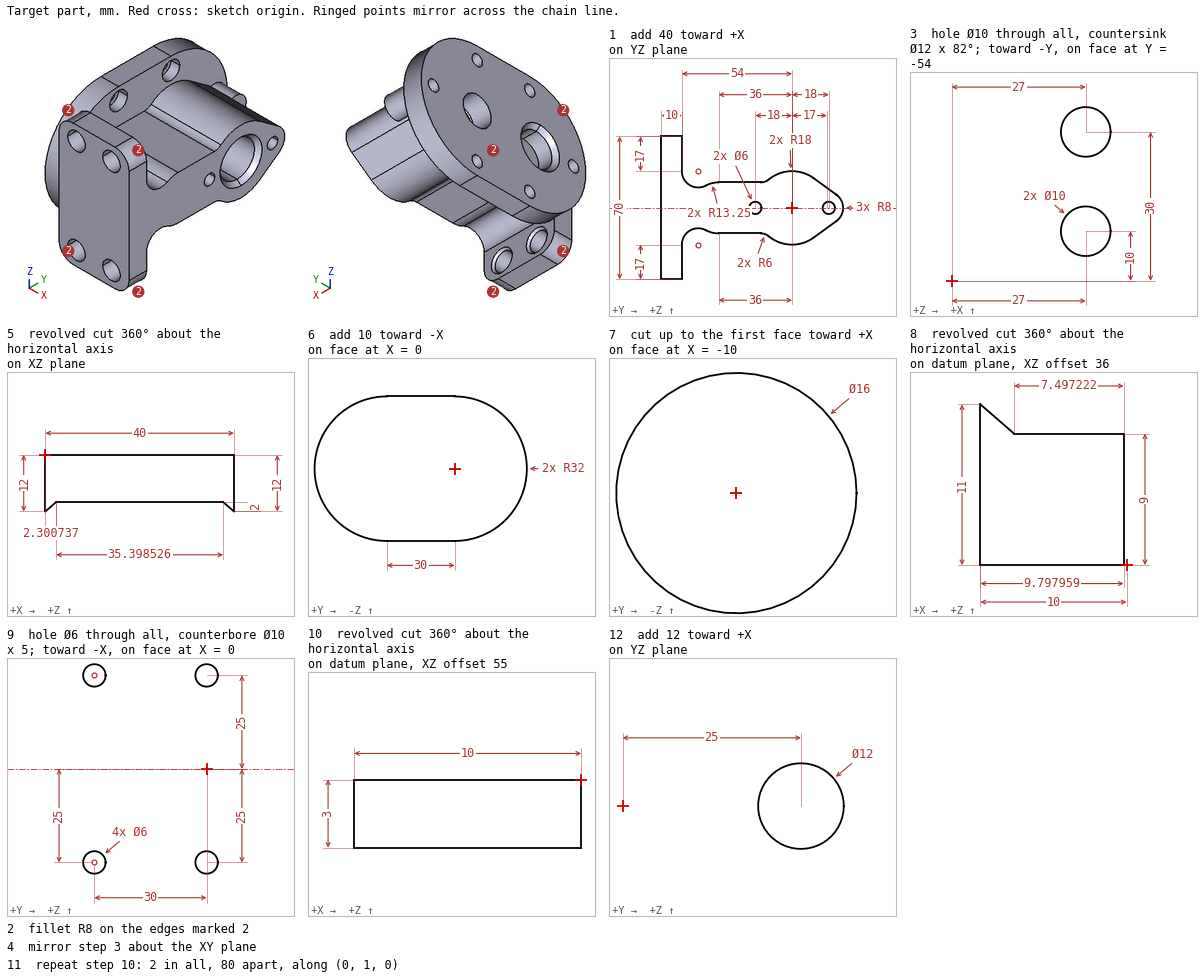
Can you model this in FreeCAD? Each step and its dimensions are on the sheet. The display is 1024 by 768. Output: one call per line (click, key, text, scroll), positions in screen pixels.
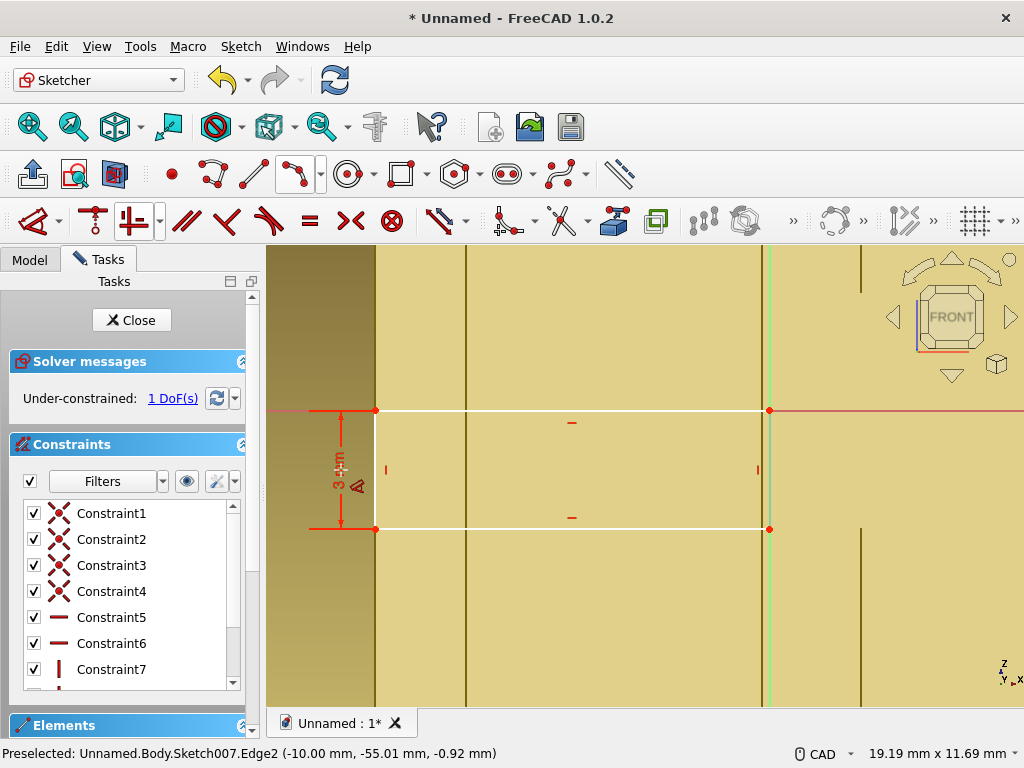
click(651, 411)
click(572, 377)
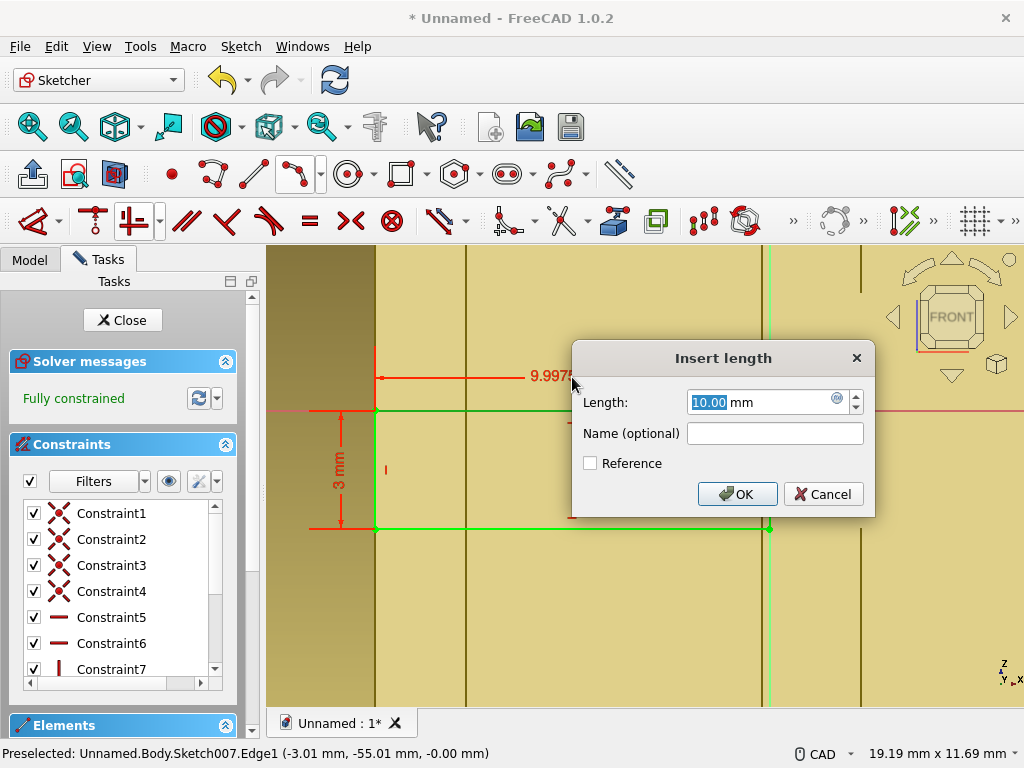
text(10)
key(Return)
key(Escape)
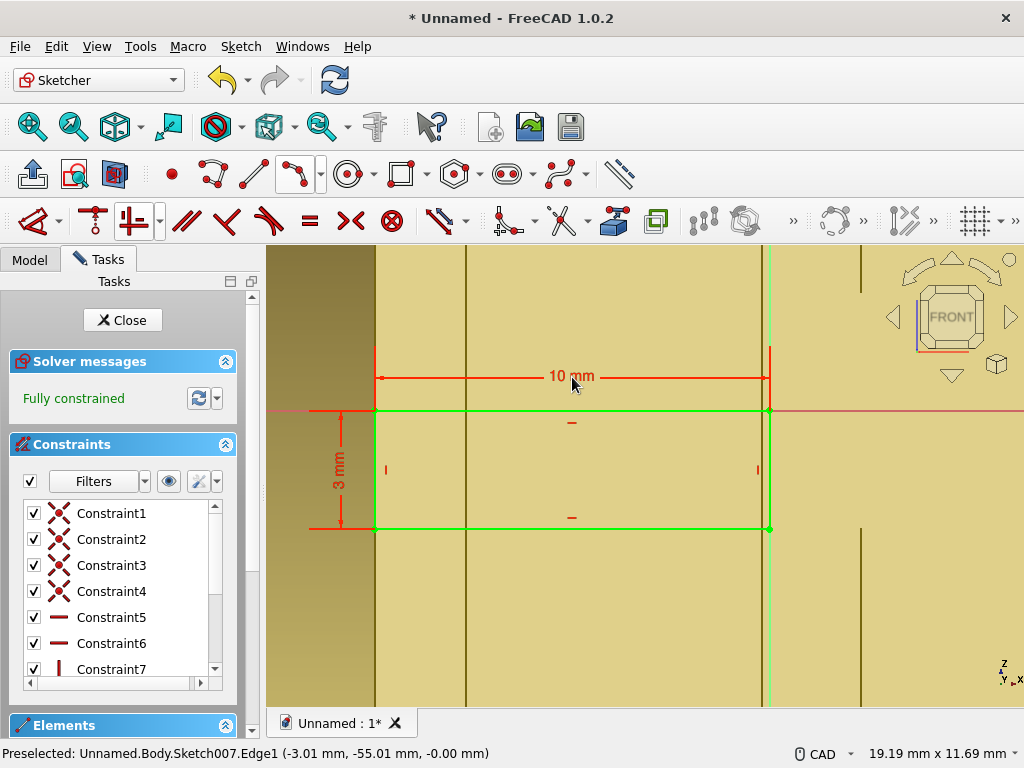
click(123, 320)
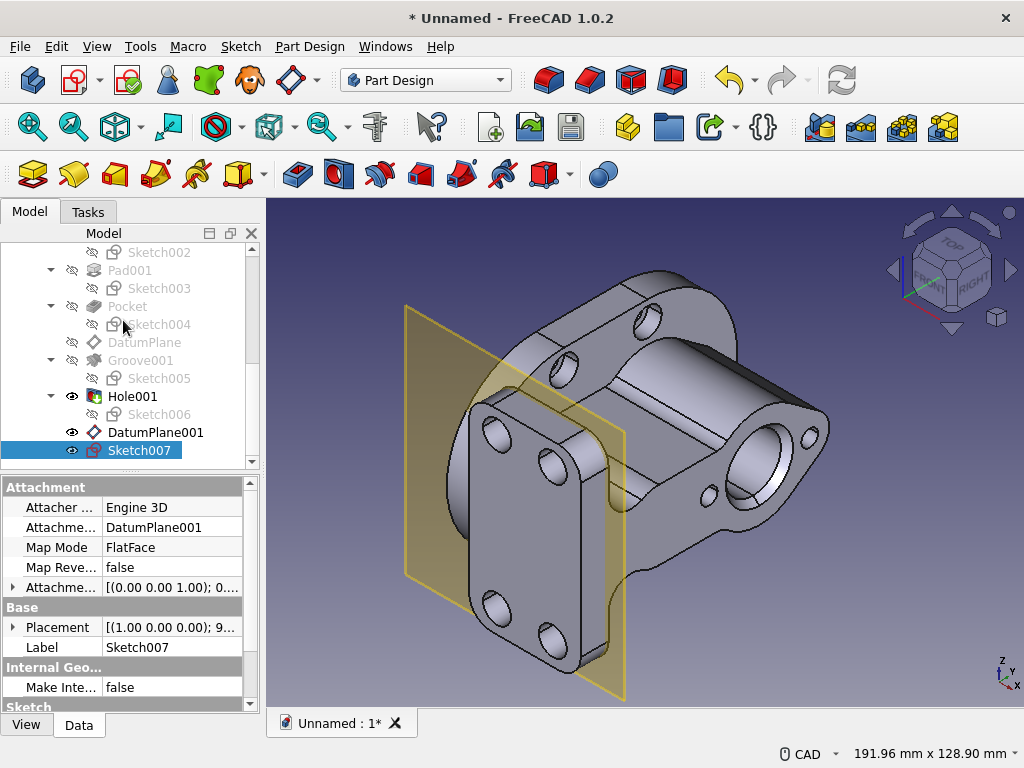
click(380, 174)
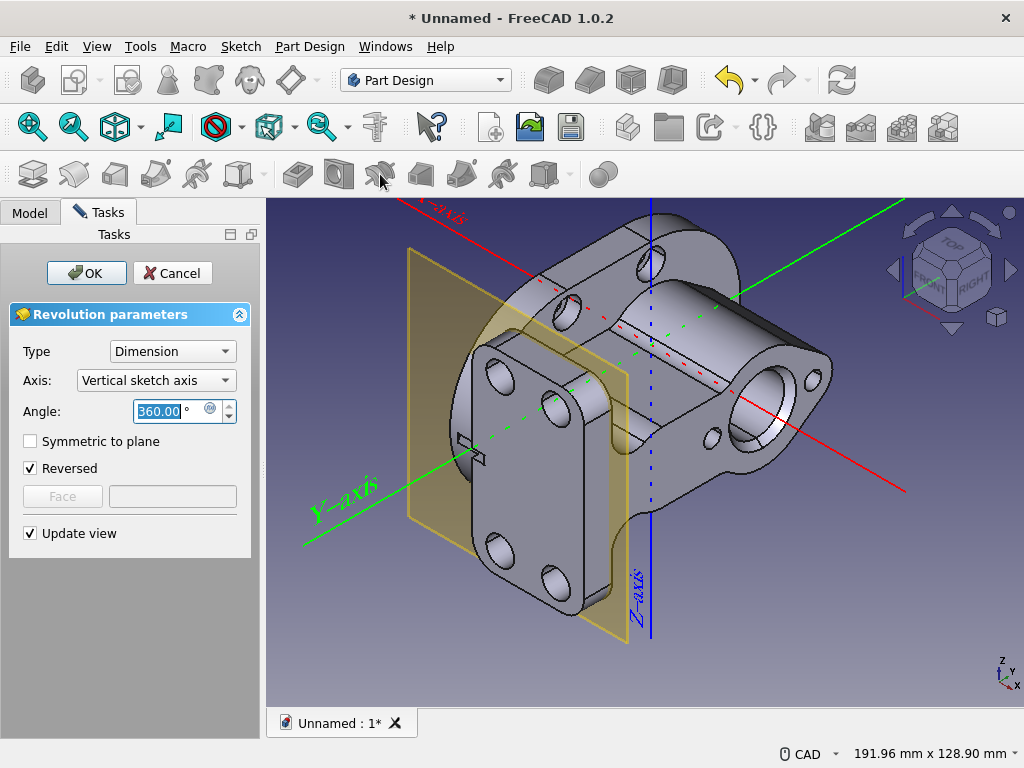
click(157, 380)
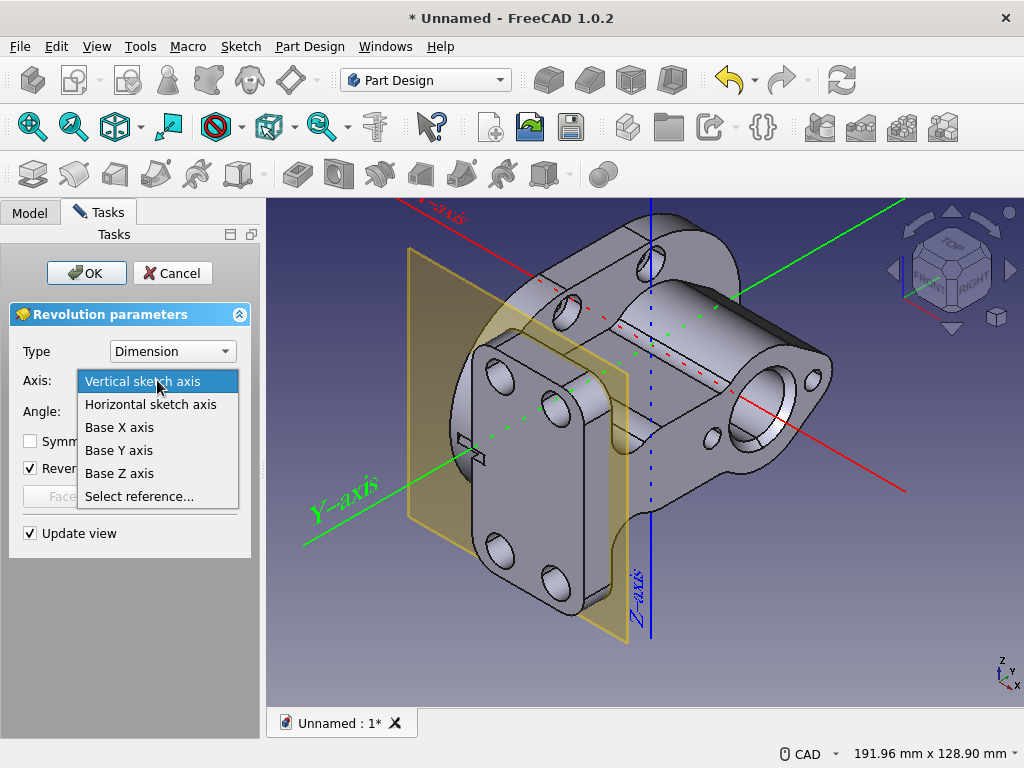
click(156, 404)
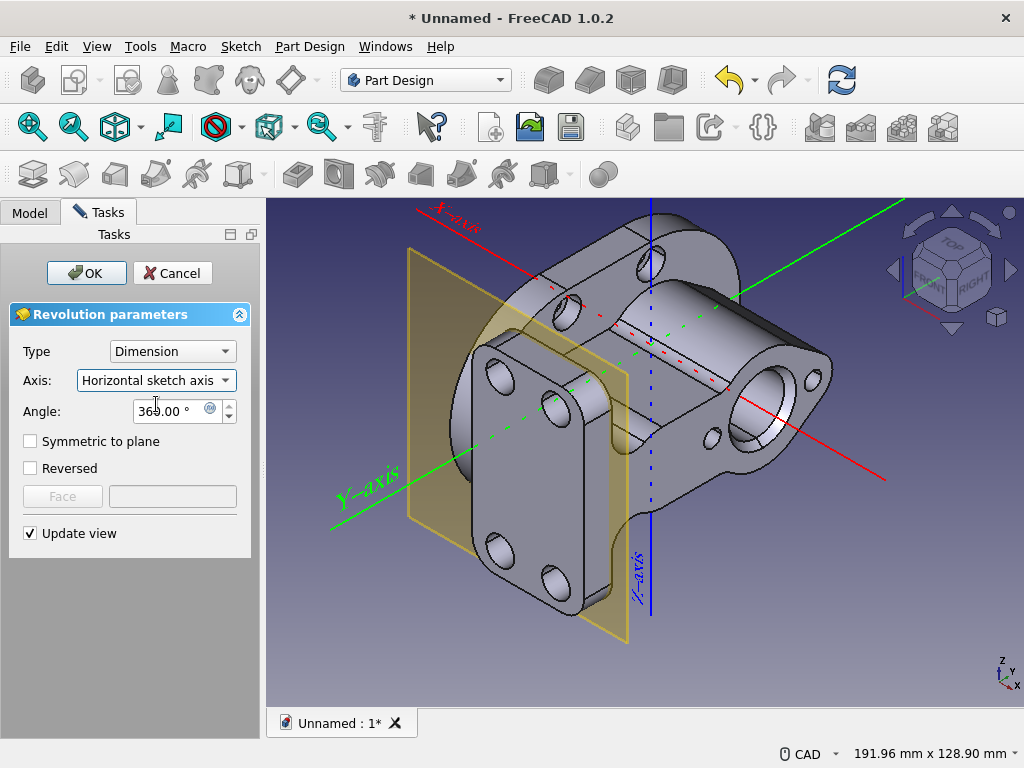
click(87, 273)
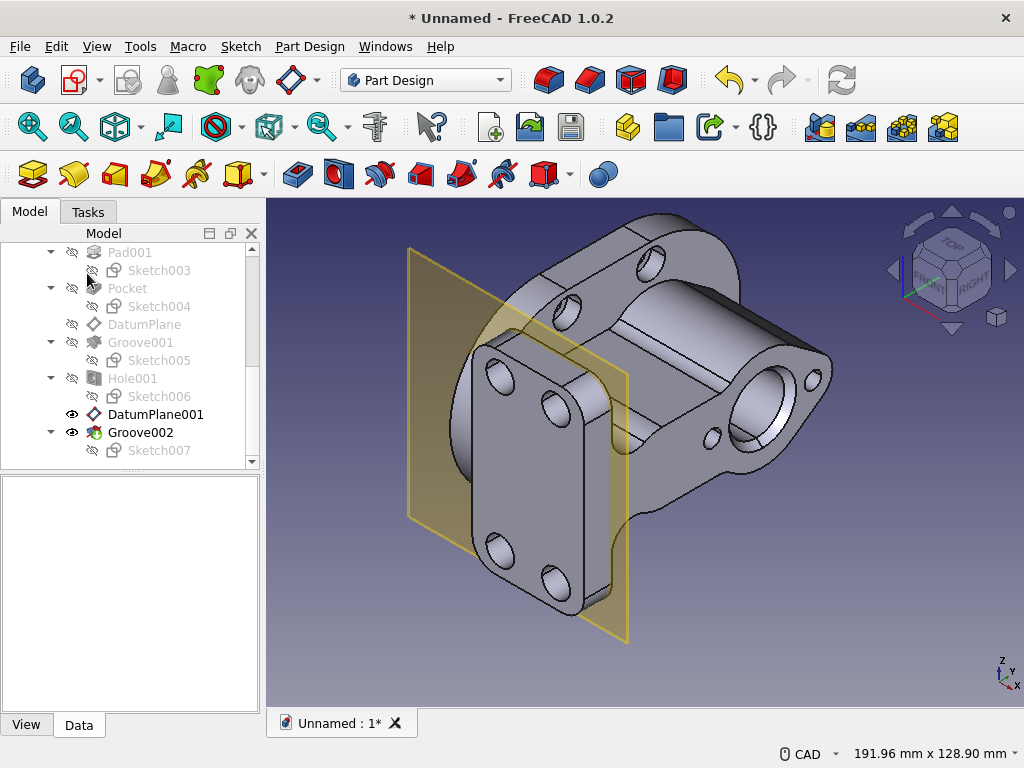
click(117, 414)
key(space)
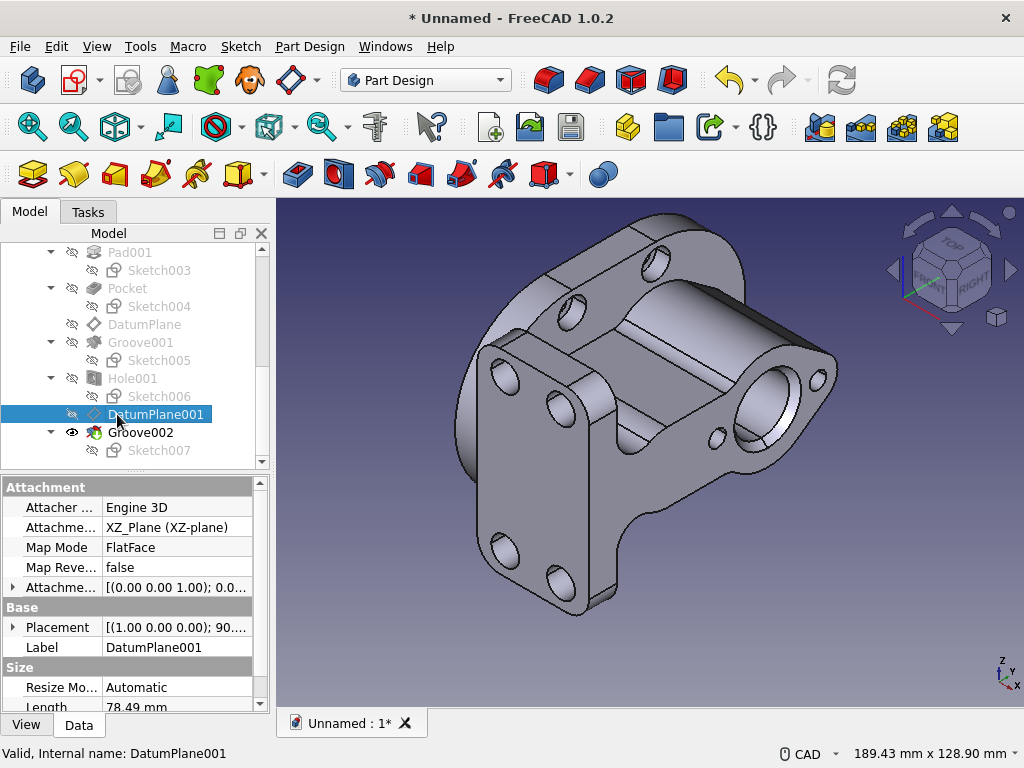
click(33, 128)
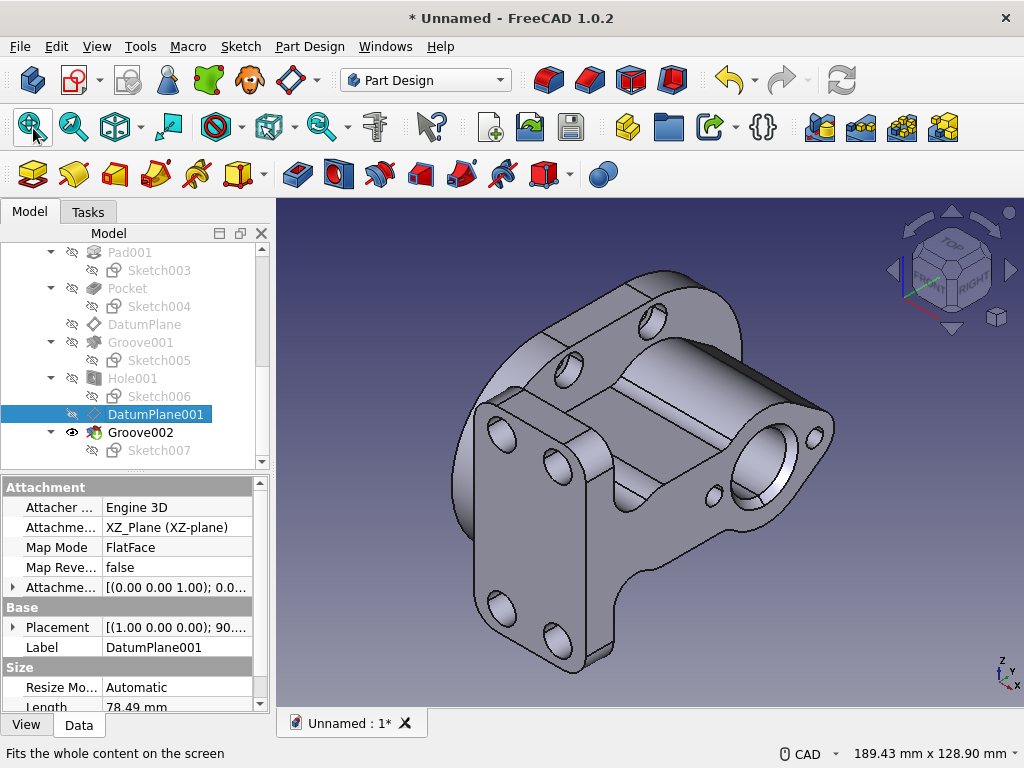
click(117, 432)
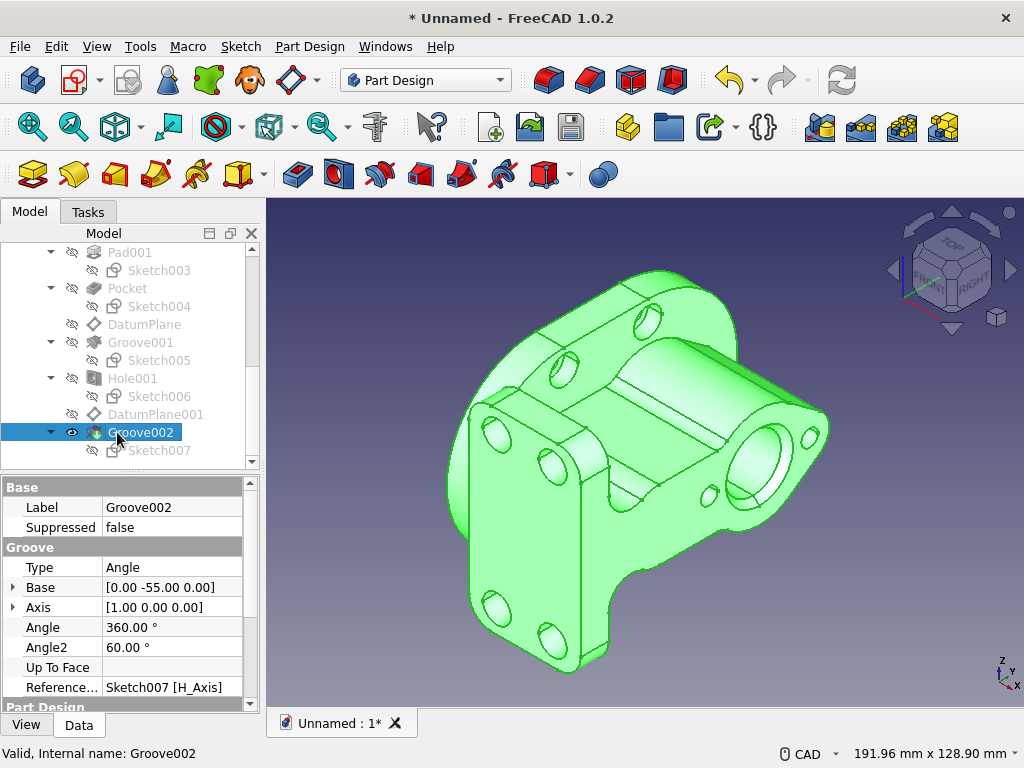
click(861, 128)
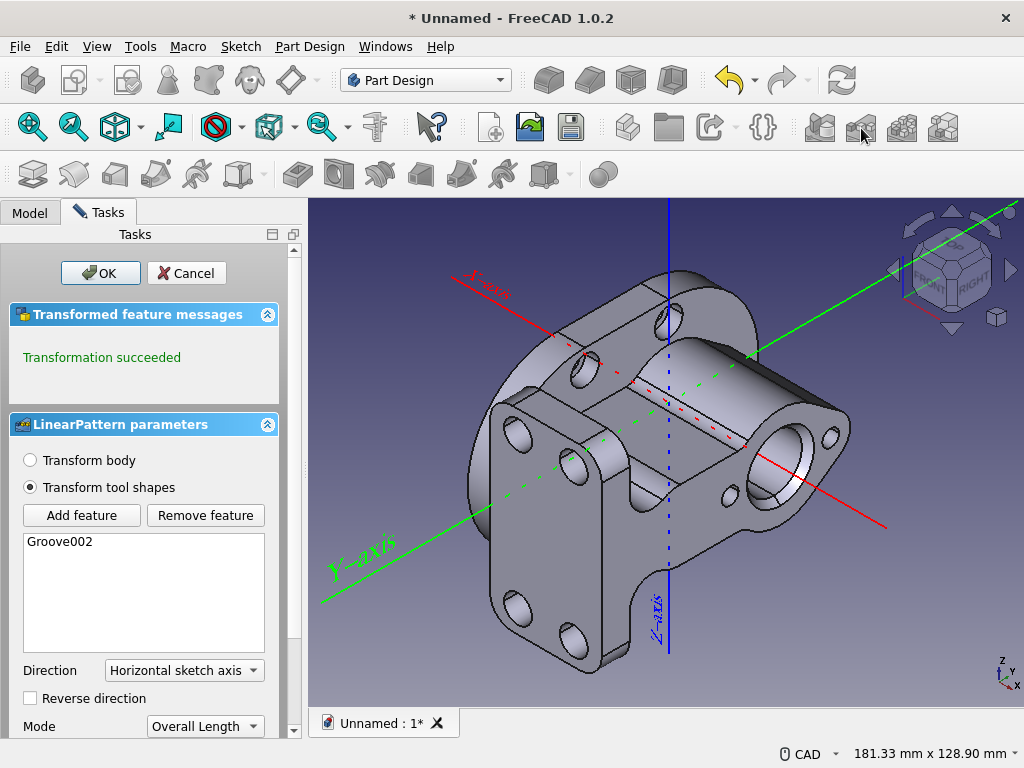
click(185, 670)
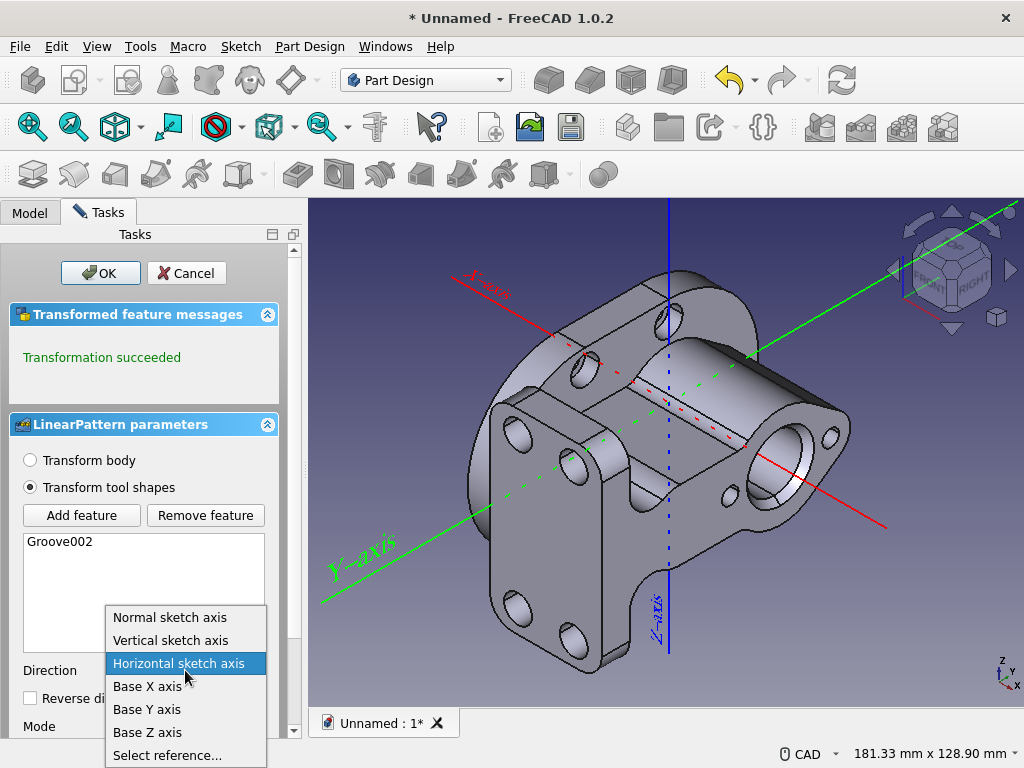
click(184, 710)